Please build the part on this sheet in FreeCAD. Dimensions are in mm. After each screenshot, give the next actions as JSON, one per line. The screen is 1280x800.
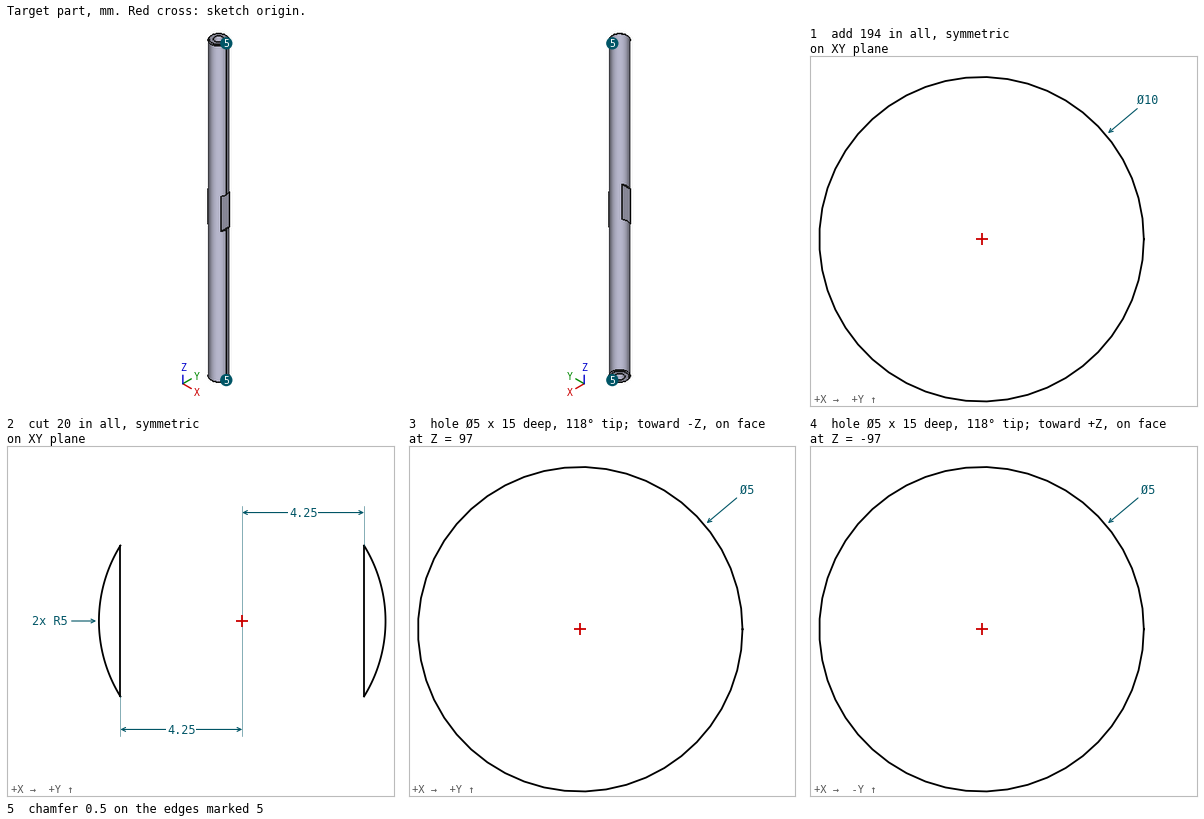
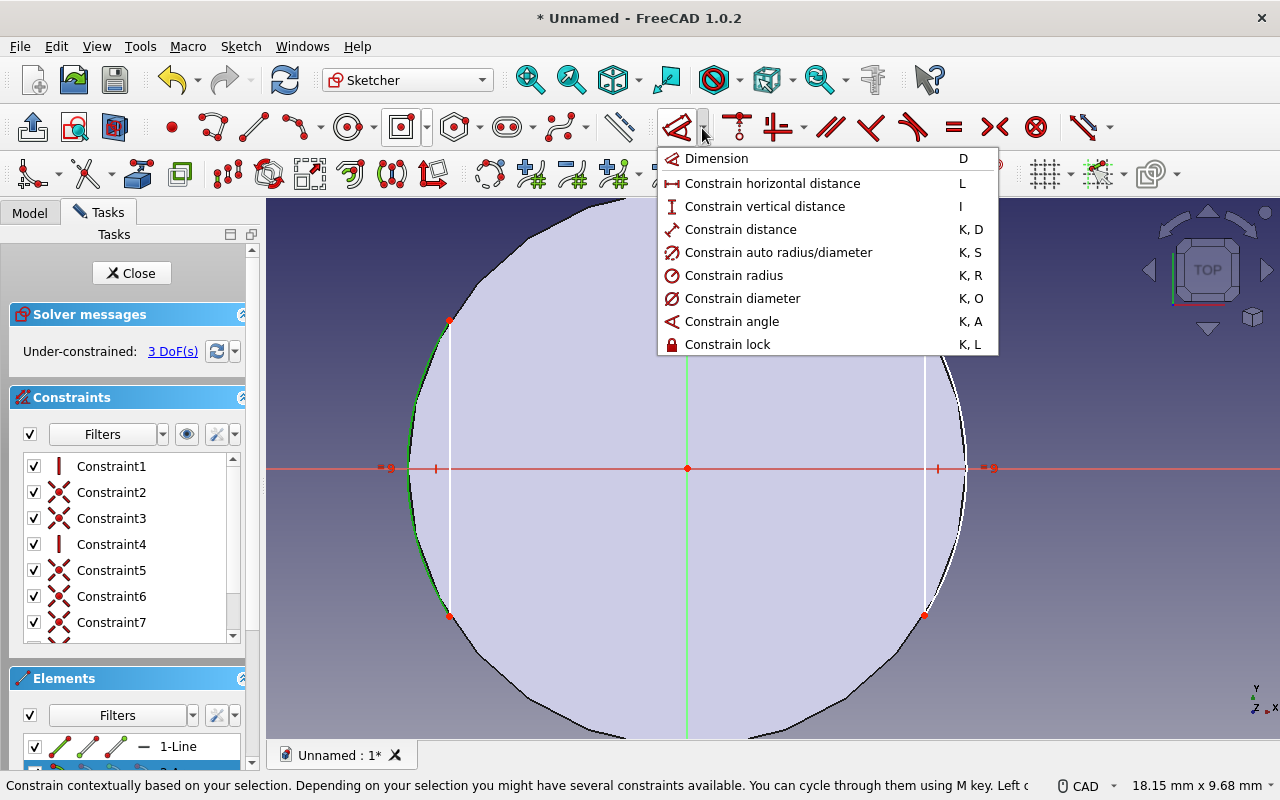
{"action": "left_click", "coordinate": [828, 276]}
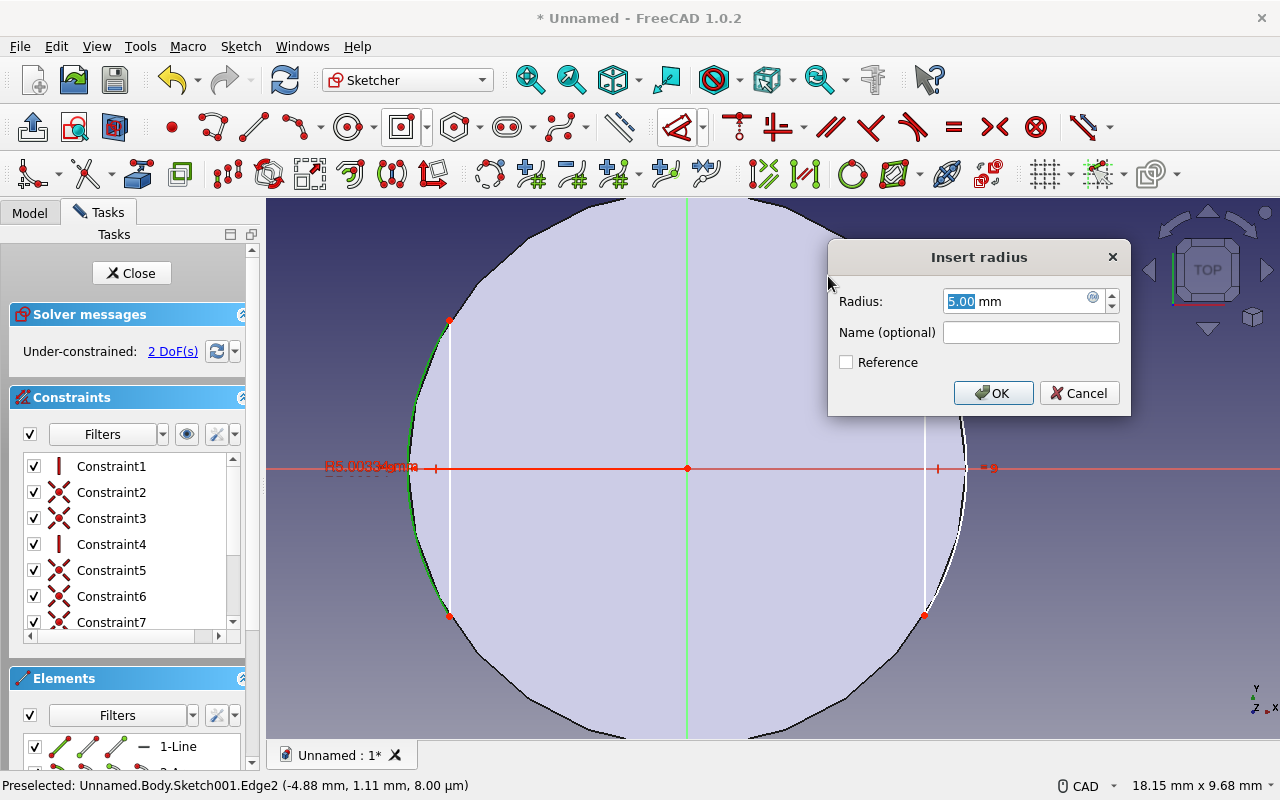
{"action": "type", "text": "5"}
{"action": "key", "text": "Return"}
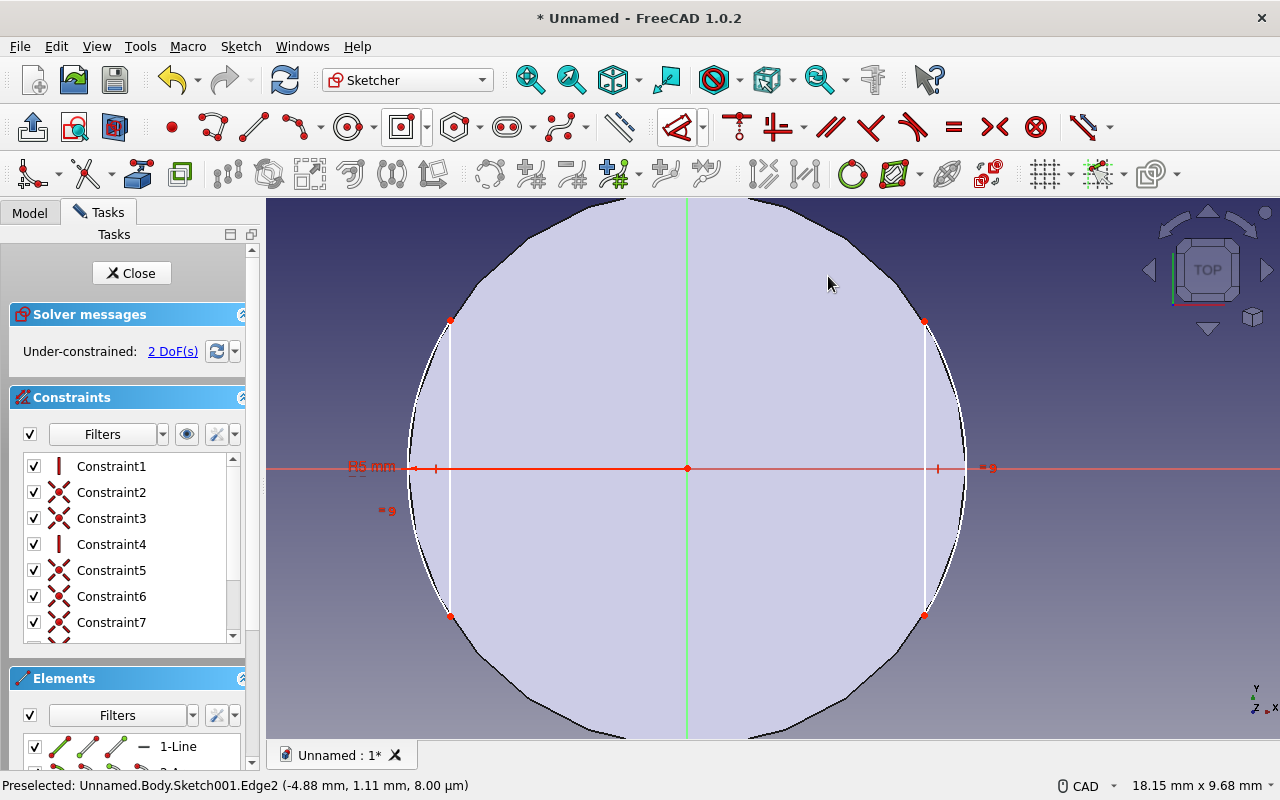
{"action": "left_click", "coordinate": [450, 617]}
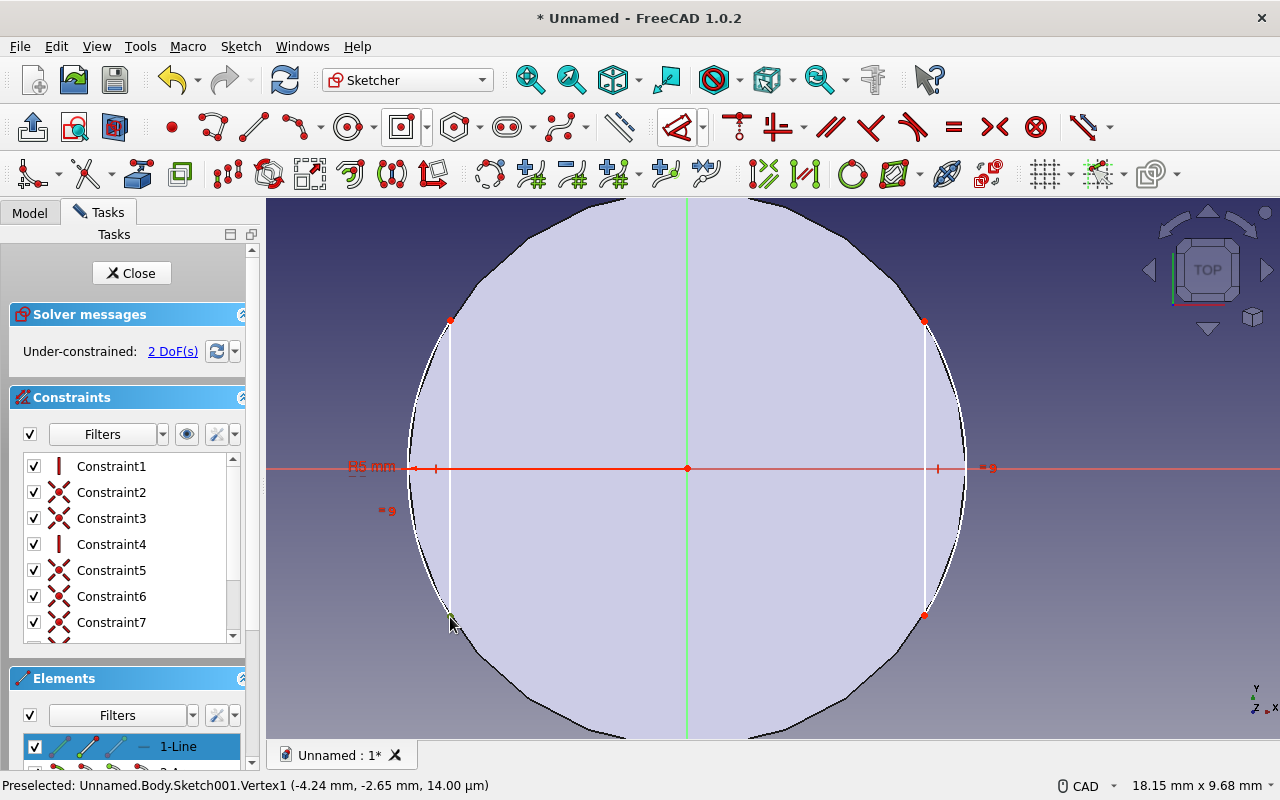
{"action": "left_click", "coordinate": [702, 128]}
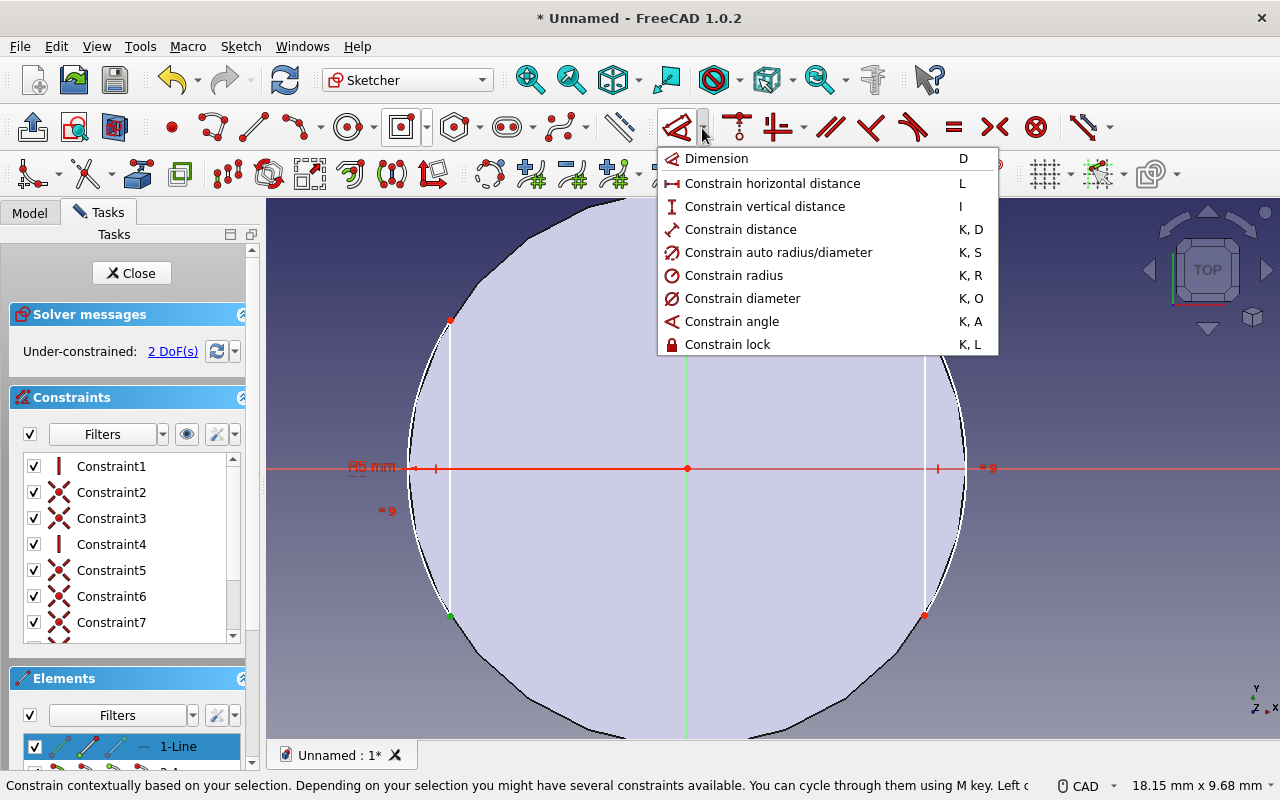
{"action": "left_click", "coordinate": [828, 184]}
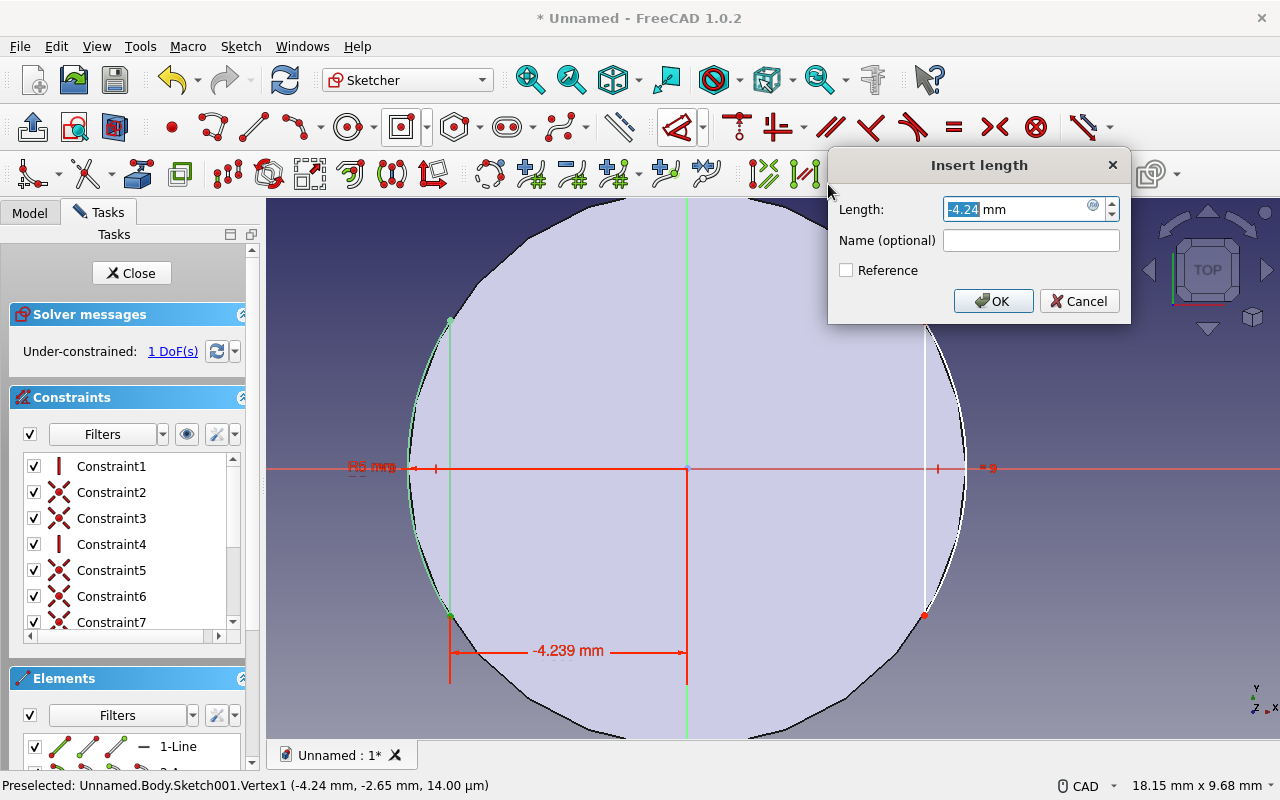
{"action": "type", "text": "-4.25"}
{"action": "key", "text": "Return"}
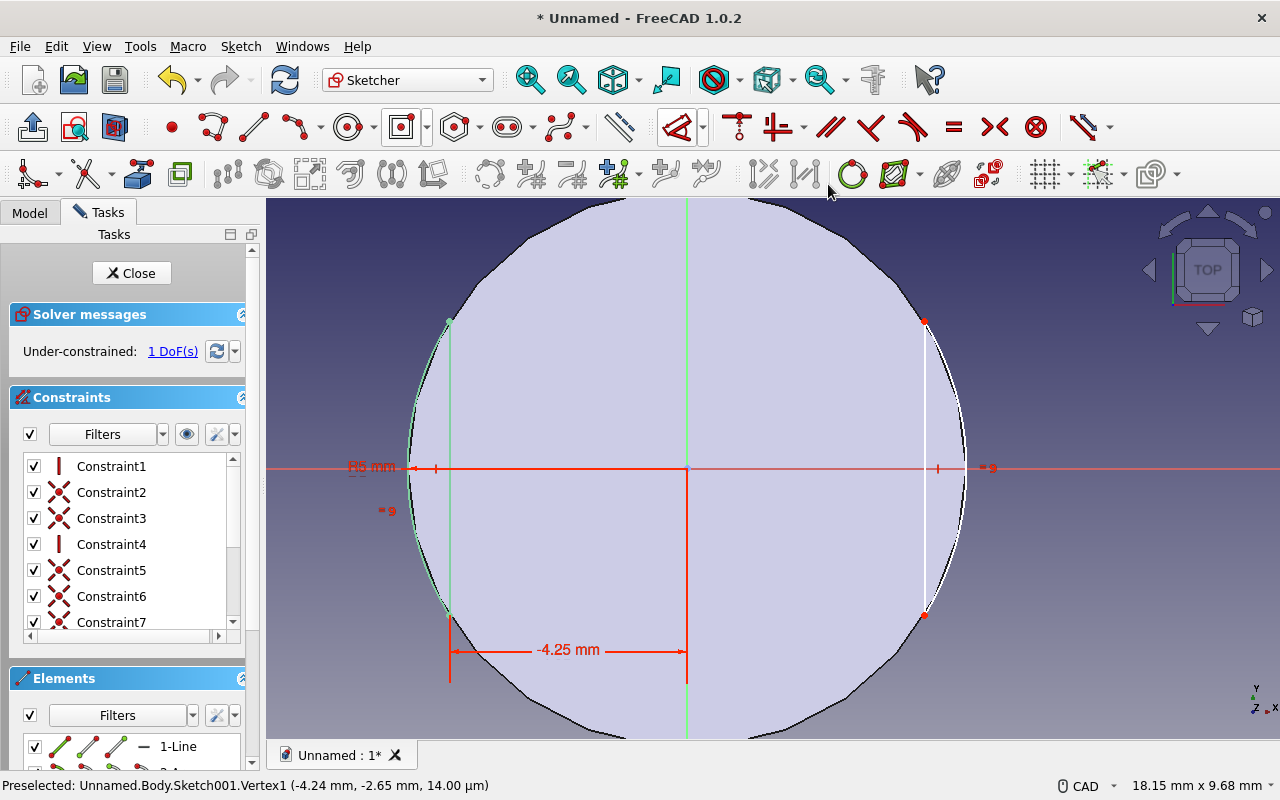
{"action": "left_click", "coordinate": [925, 322]}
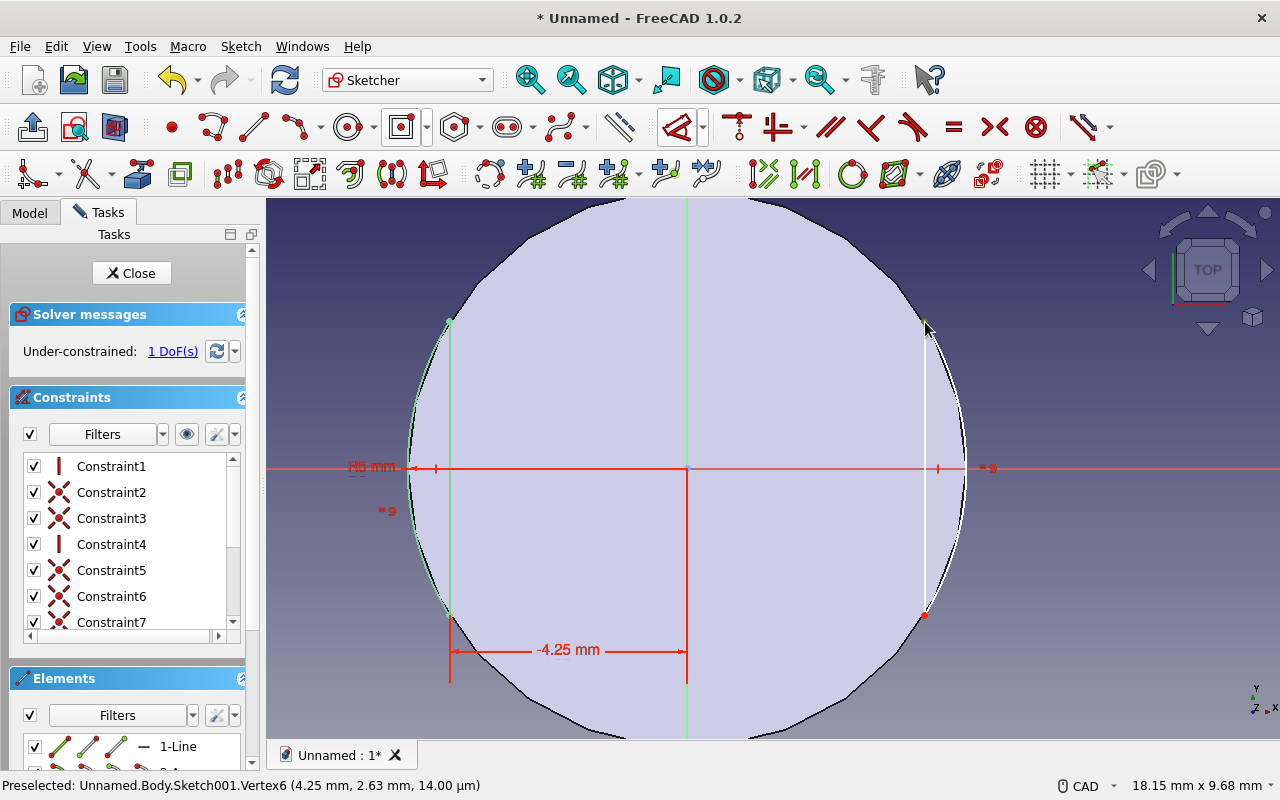
{"action": "left_click", "coordinate": [702, 128]}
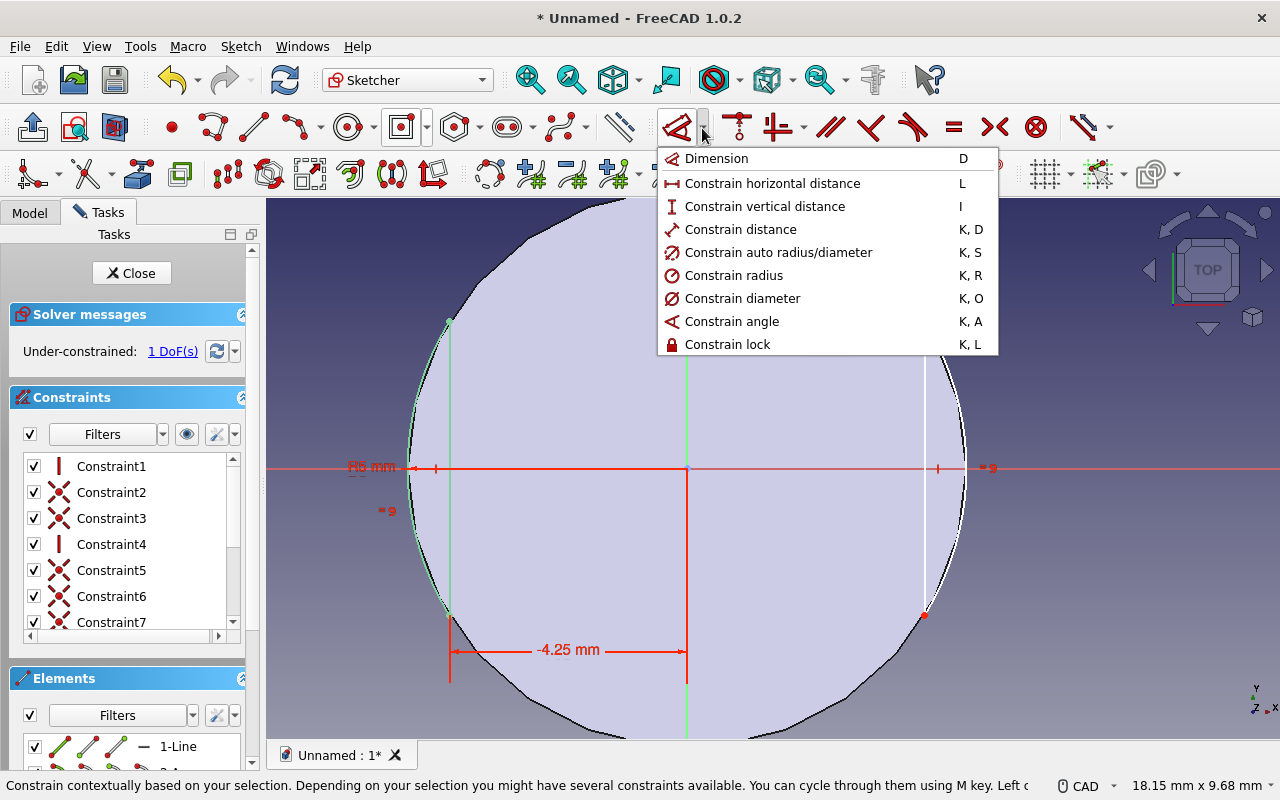
{"action": "left_click", "coordinate": [828, 184]}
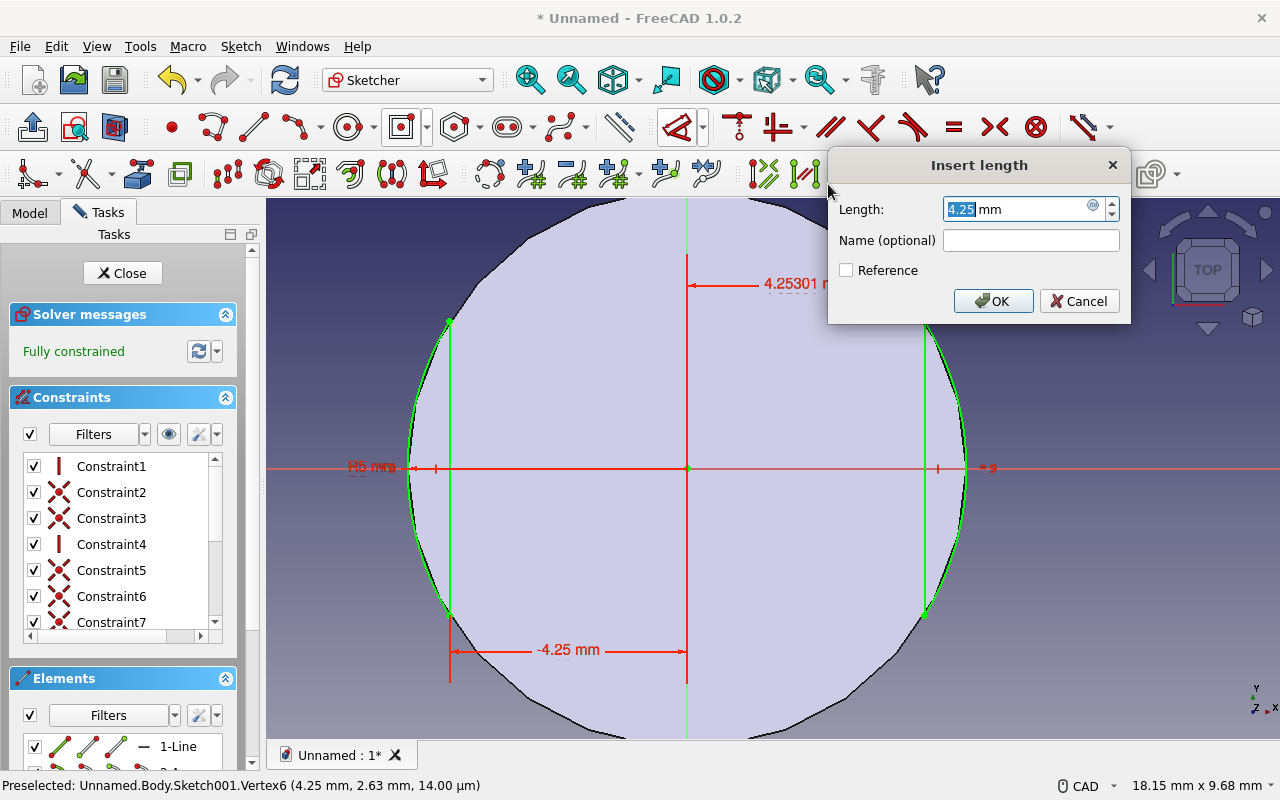
{"action": "type", "text": "4.25"}
{"action": "key", "text": "Return"}